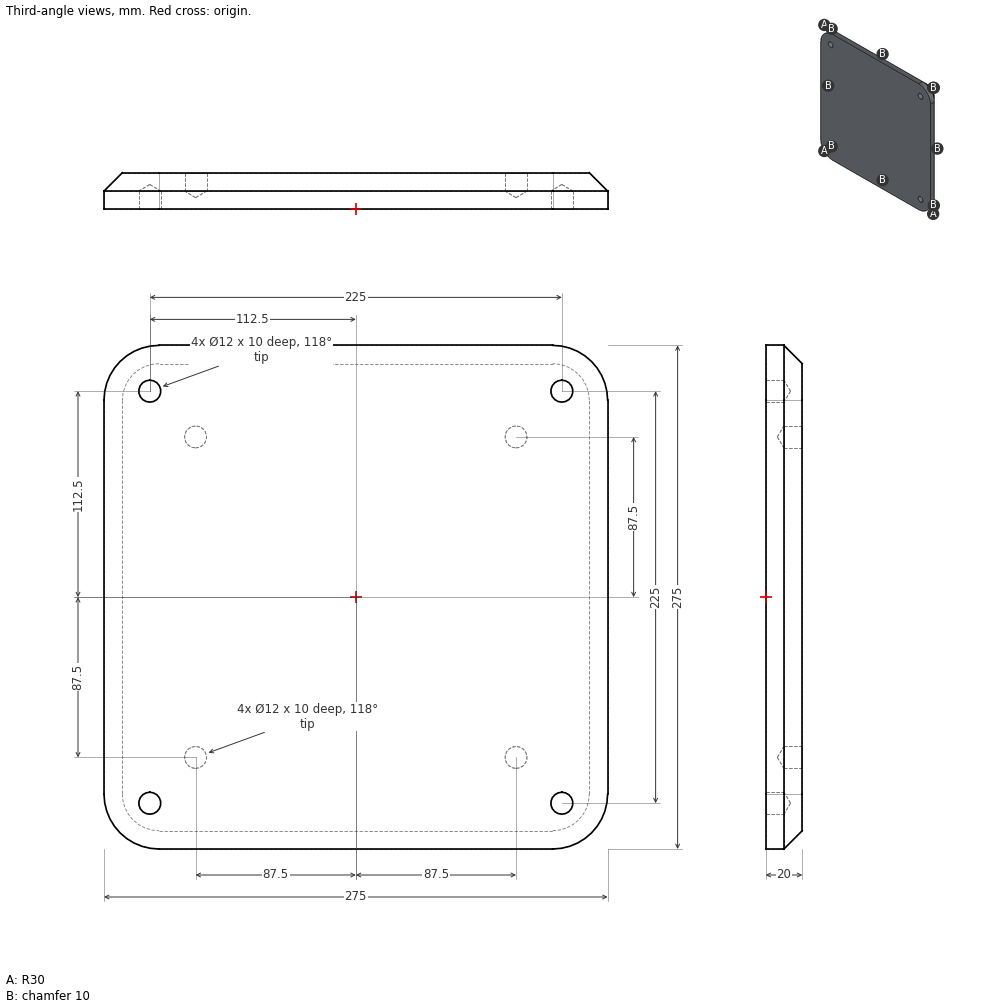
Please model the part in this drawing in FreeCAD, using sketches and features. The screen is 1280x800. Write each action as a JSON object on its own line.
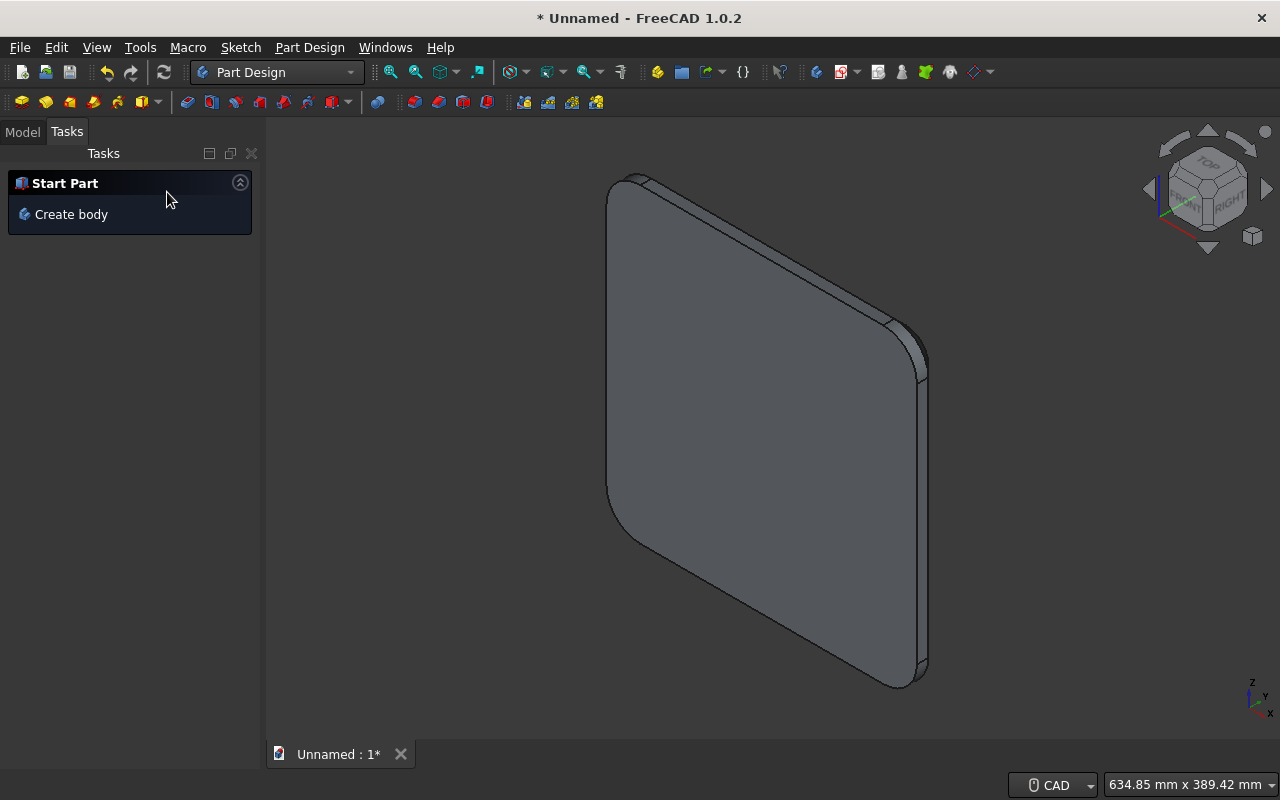
{"action": "left_click", "coordinate": [762, 434]}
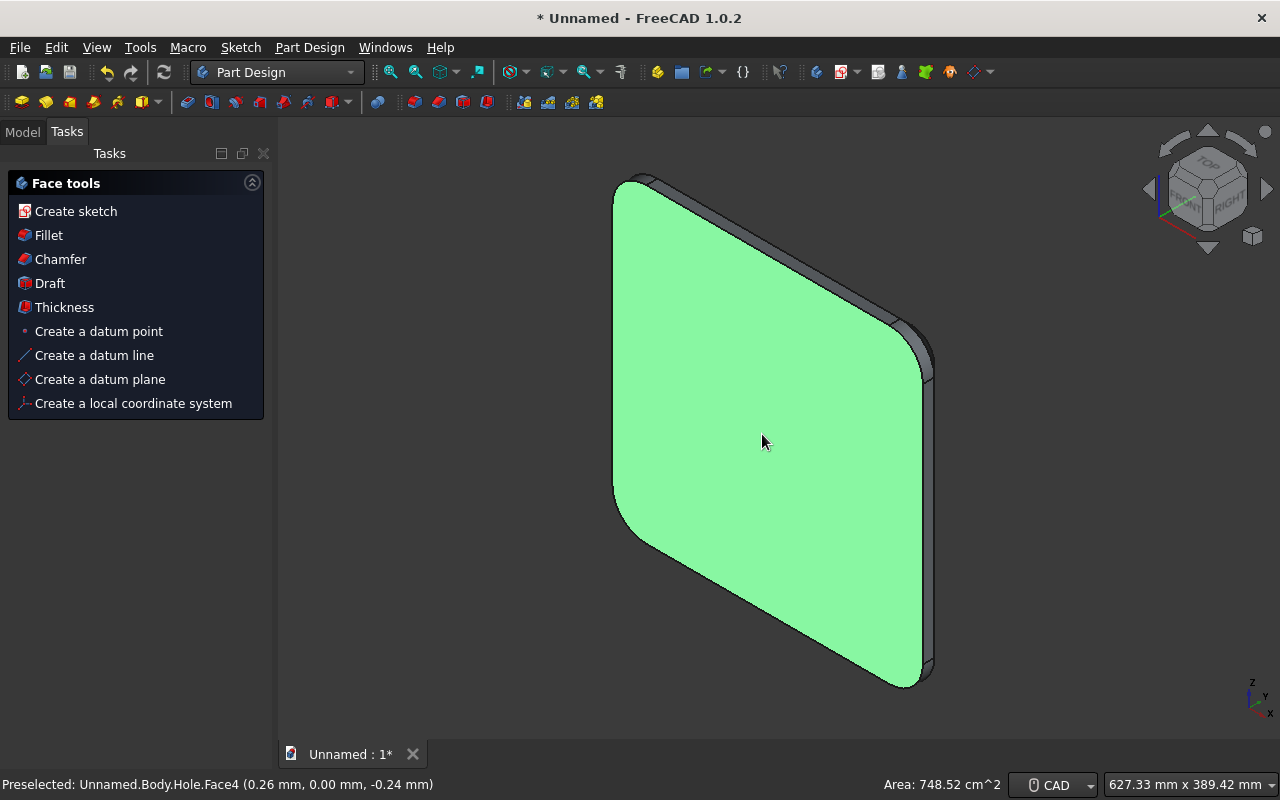
{"action": "left_click", "coordinate": [842, 72]}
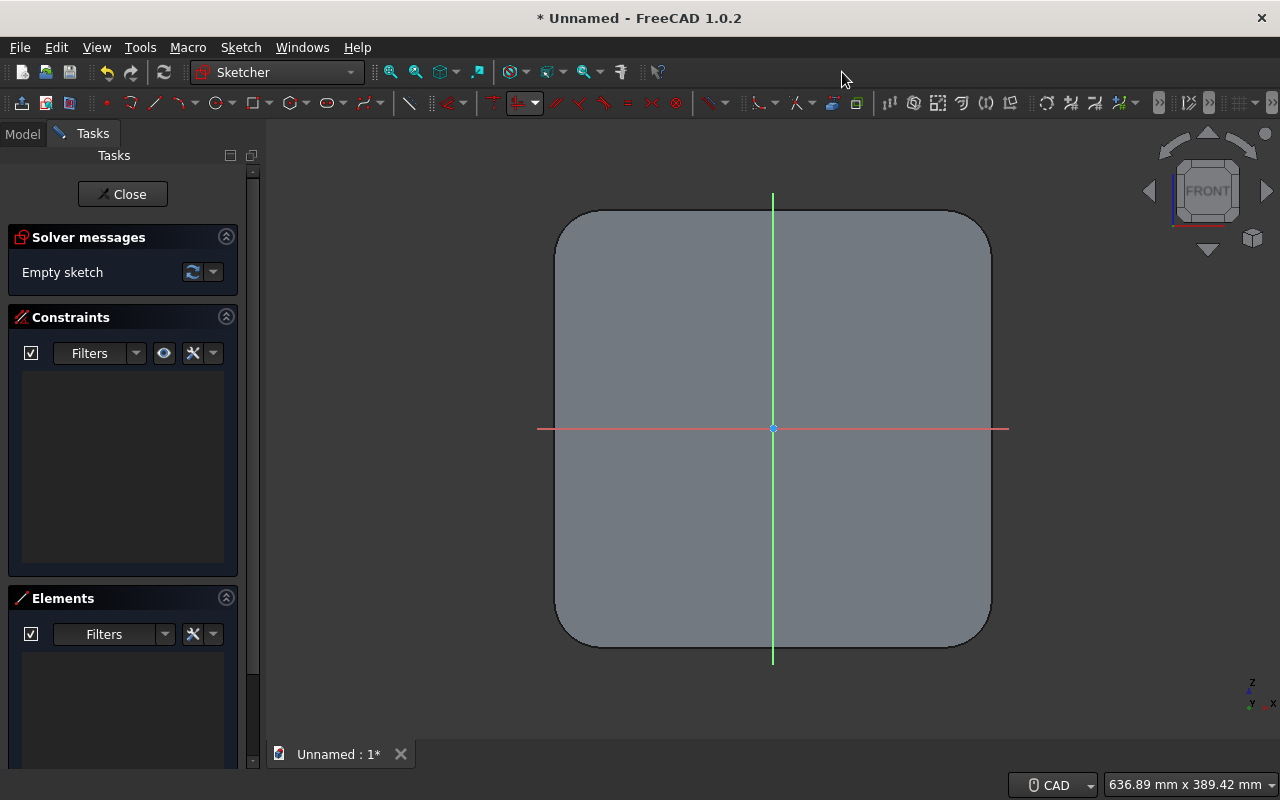
{"action": "key", "text": "g c"}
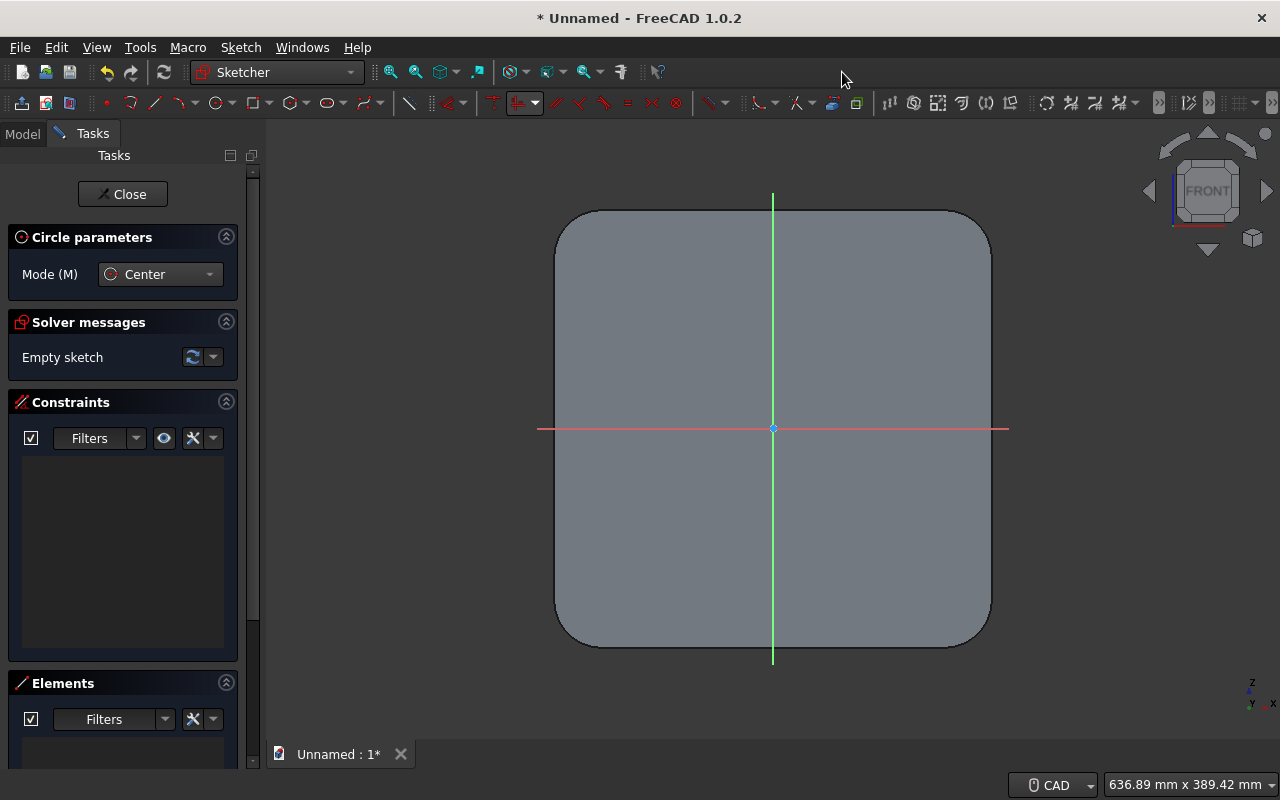
{"action": "scroll", "coordinate": [594, 250], "scroll_direction": "up", "scroll_amount": 5}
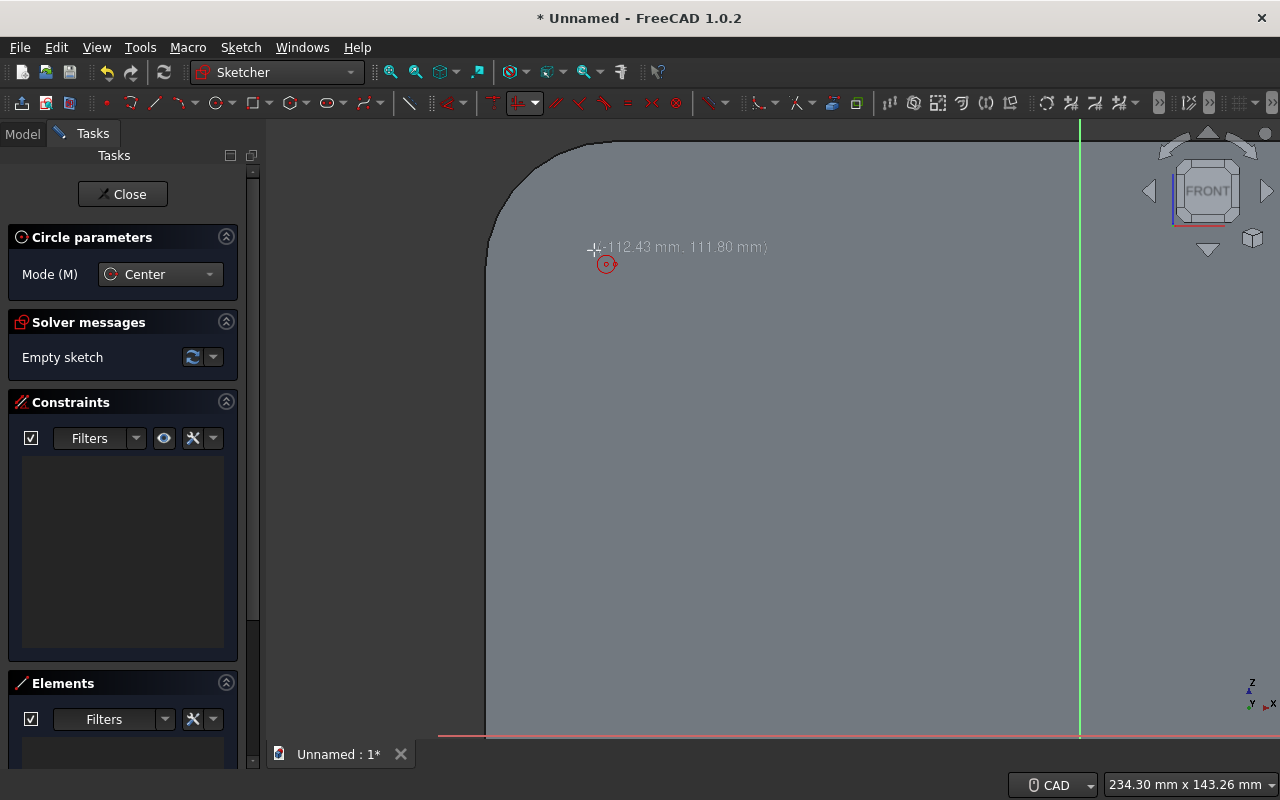
{"action": "left_click", "coordinate": [593, 249]}
{"action": "mouse_move", "coordinate": [612, 231]}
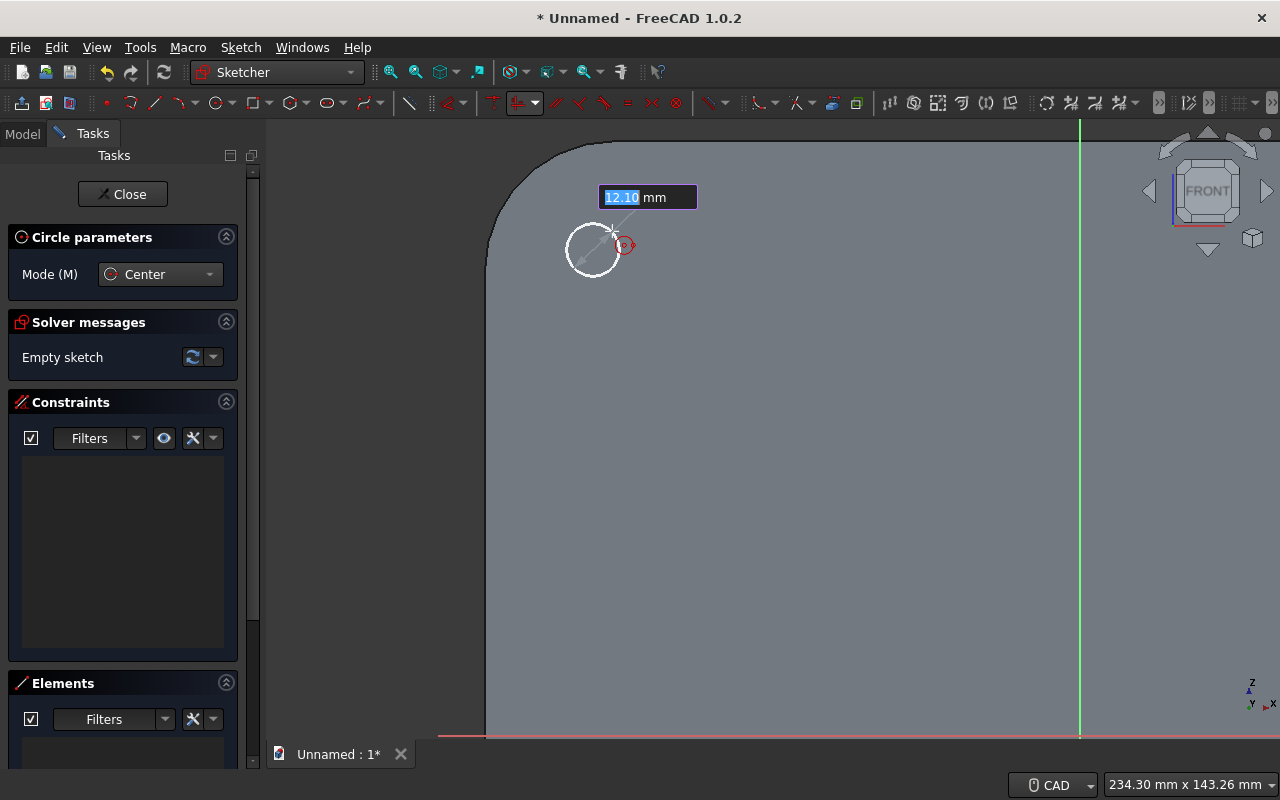
{"action": "type", "text": "12"}
{"action": "key", "text": "Return"}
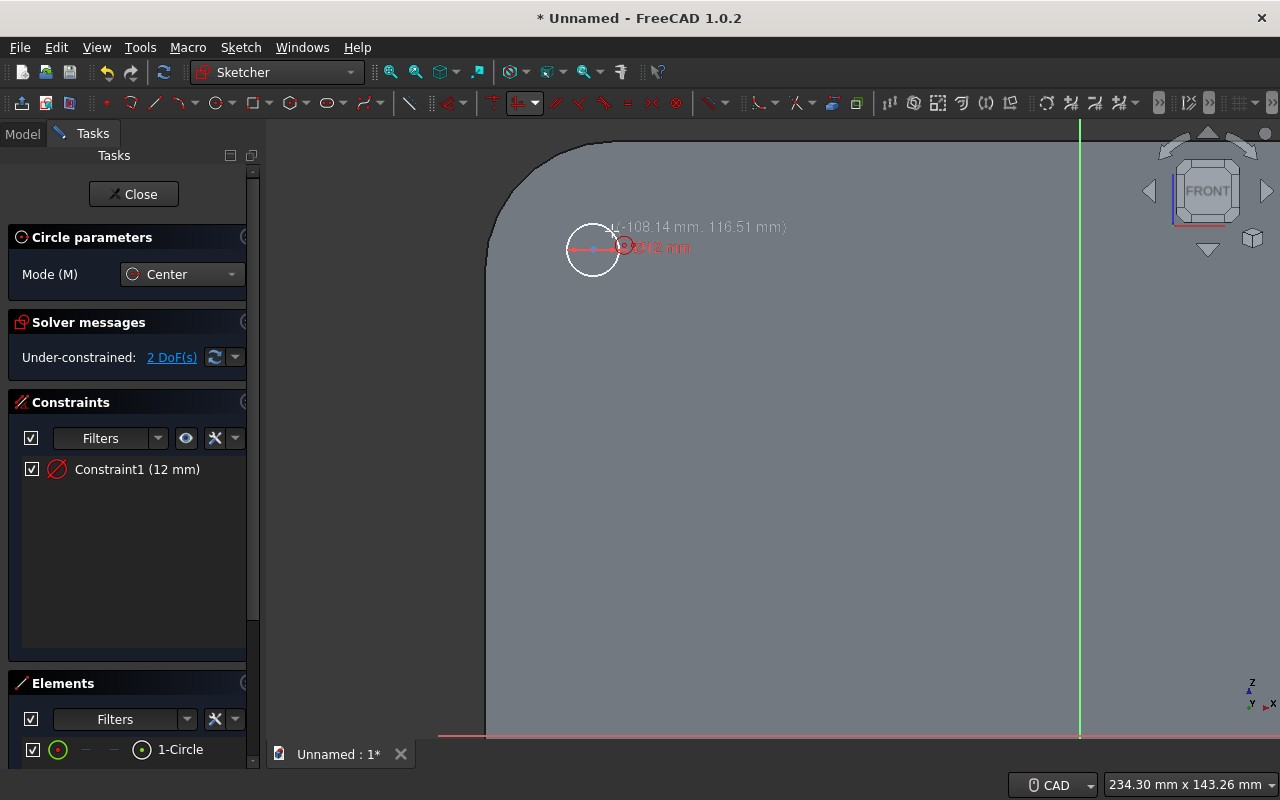
{"action": "scroll", "coordinate": [486, 250], "scroll_direction": "down", "scroll_amount": 5}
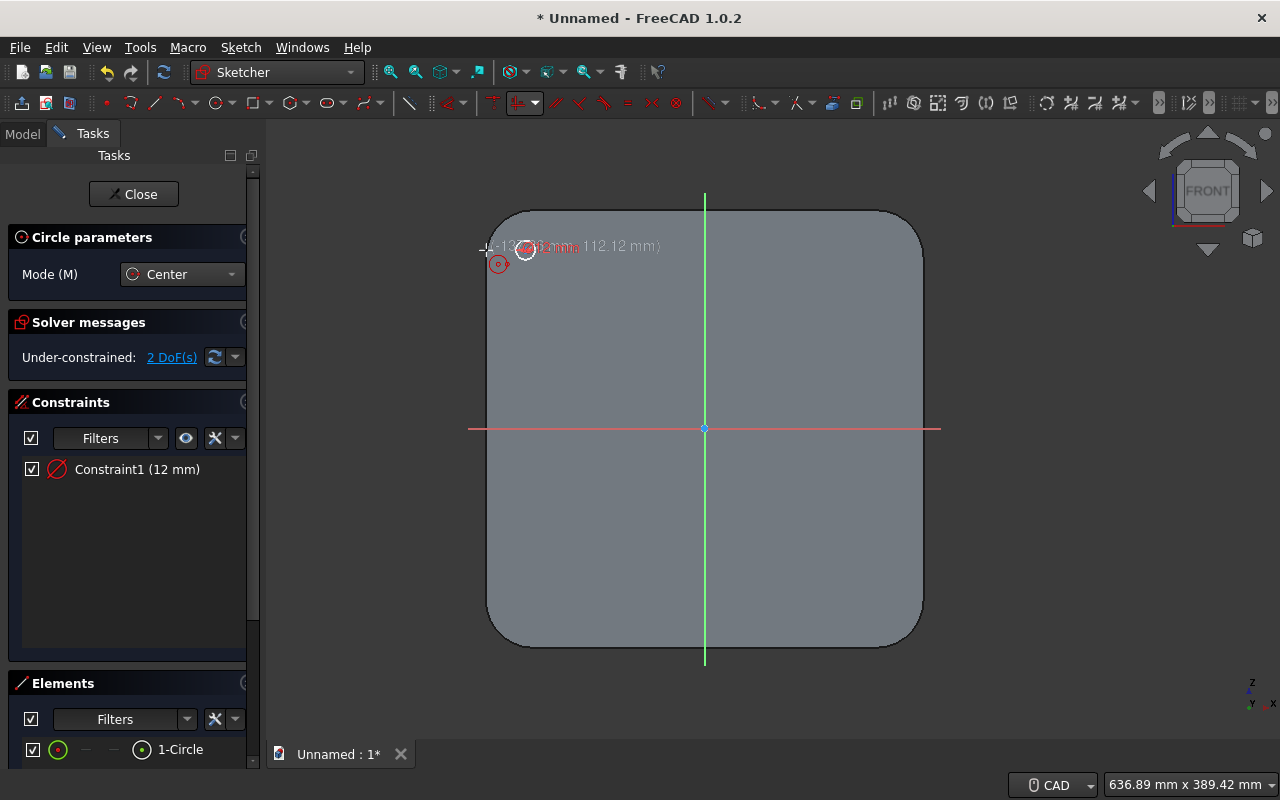
{"action": "scroll", "coordinate": [884, 250], "scroll_direction": "up", "scroll_amount": 5}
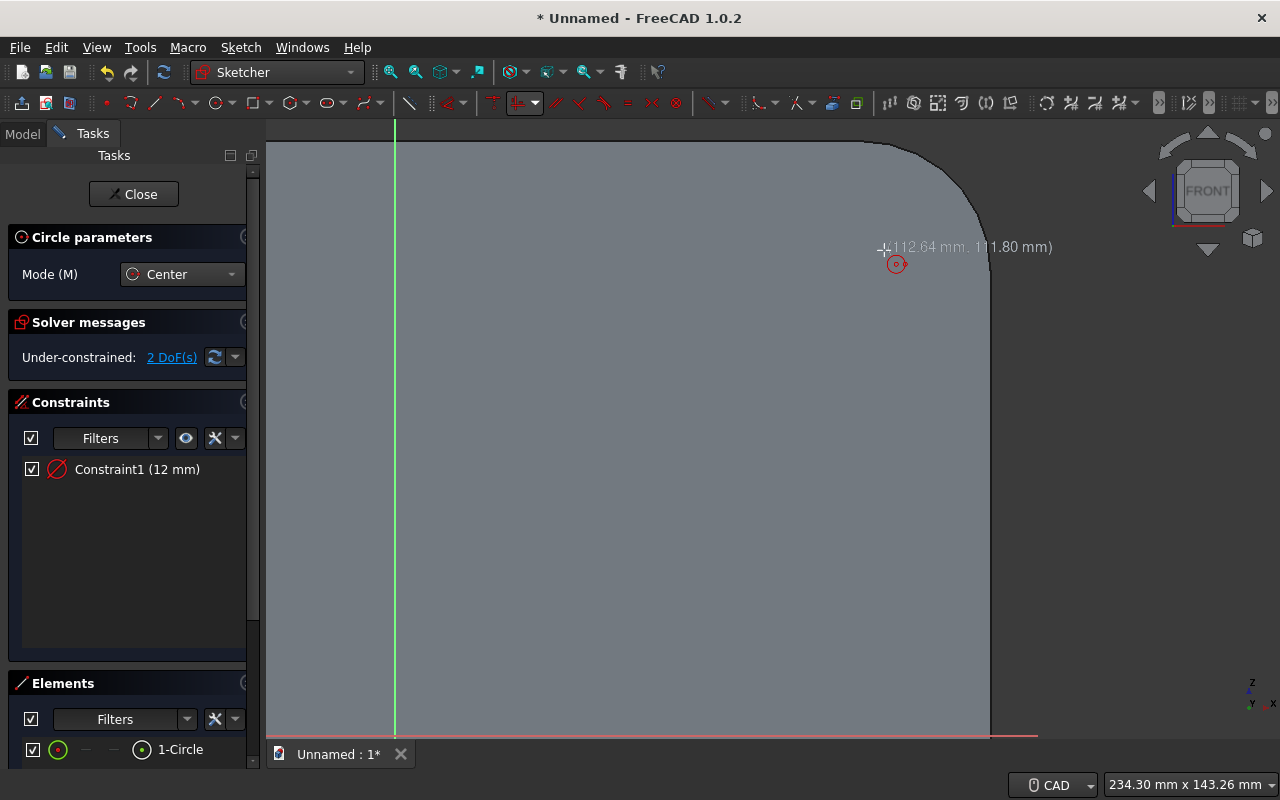
{"action": "left_click", "coordinate": [882, 249]}
{"action": "mouse_move", "coordinate": [901, 231]}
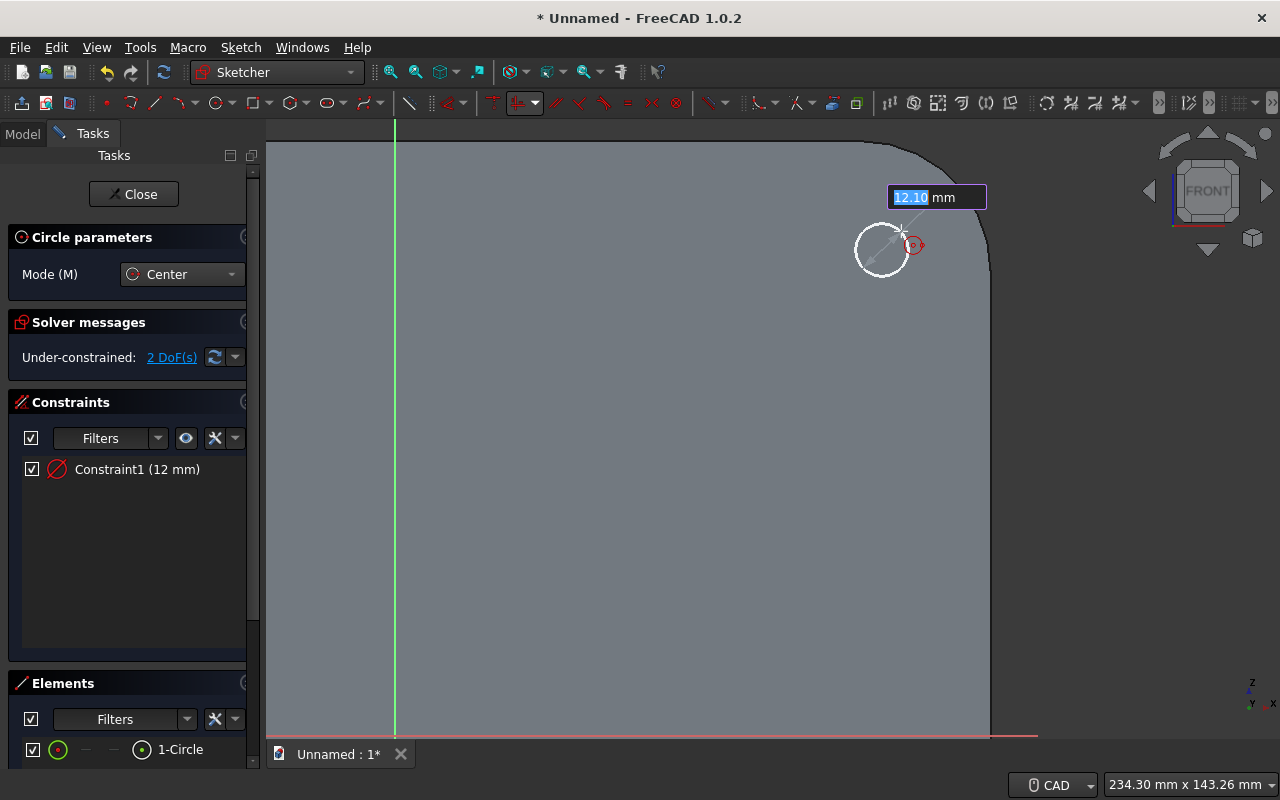
{"action": "type", "text": "12"}
{"action": "key", "text": "Return"}